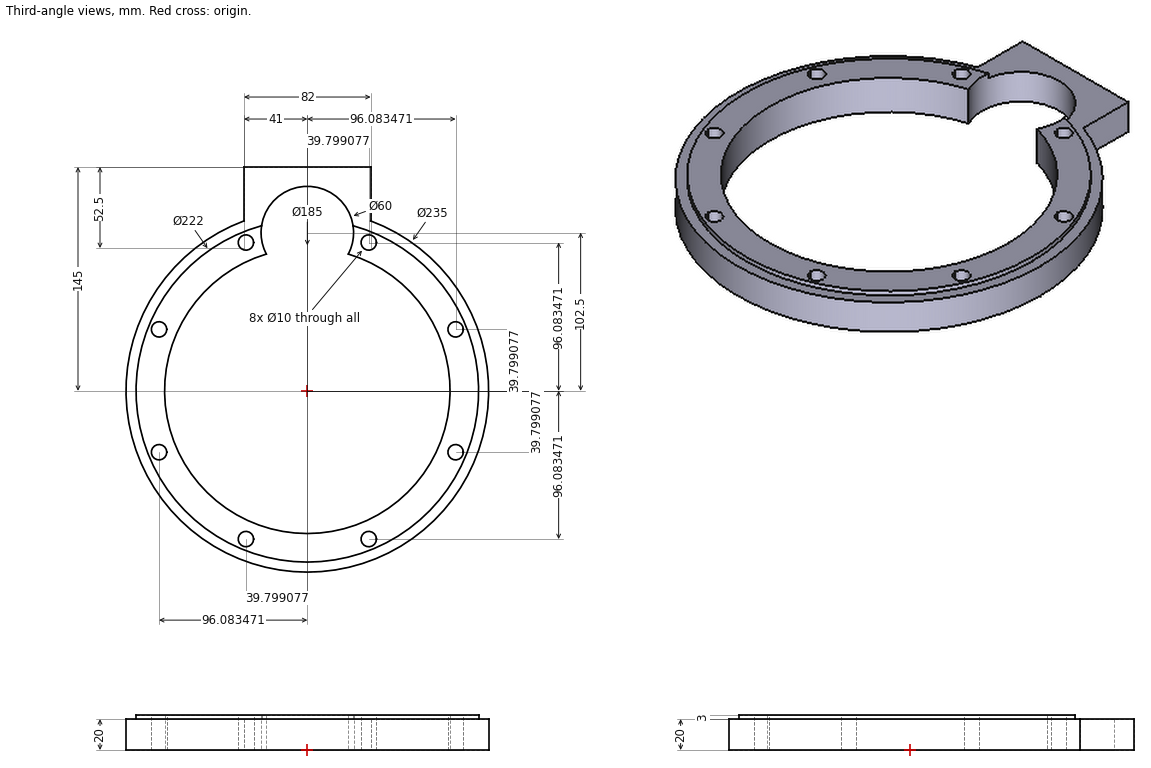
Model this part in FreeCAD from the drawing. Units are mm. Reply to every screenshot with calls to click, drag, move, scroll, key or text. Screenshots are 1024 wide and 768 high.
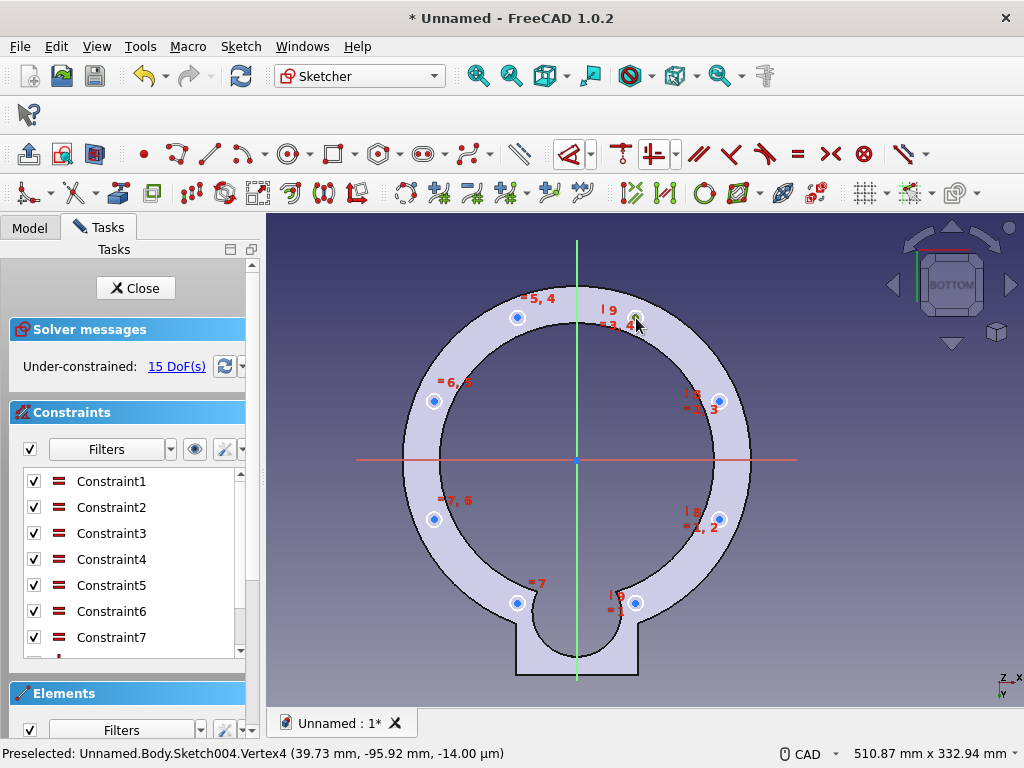
click(518, 318)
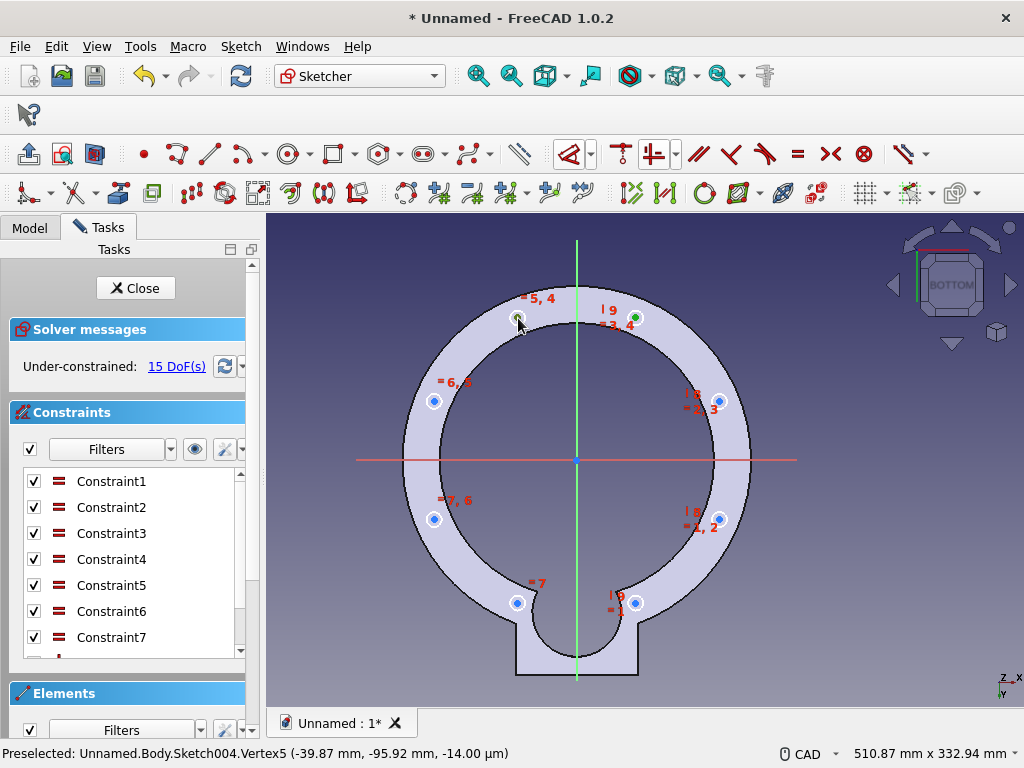
click(676, 154)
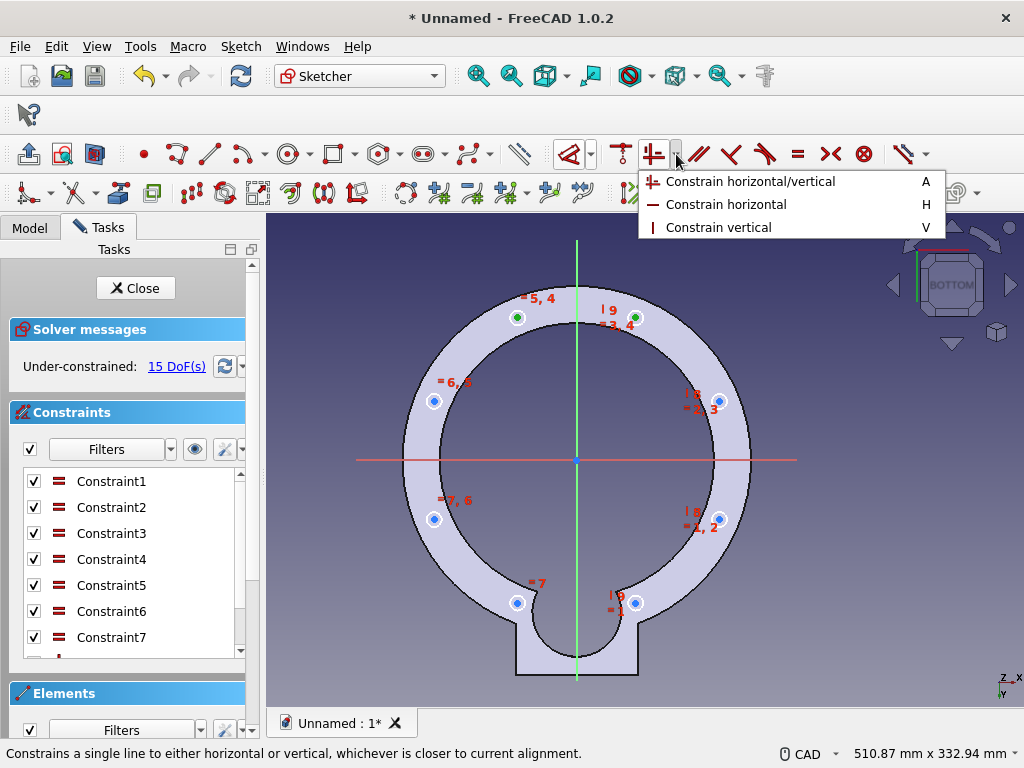
click(792, 204)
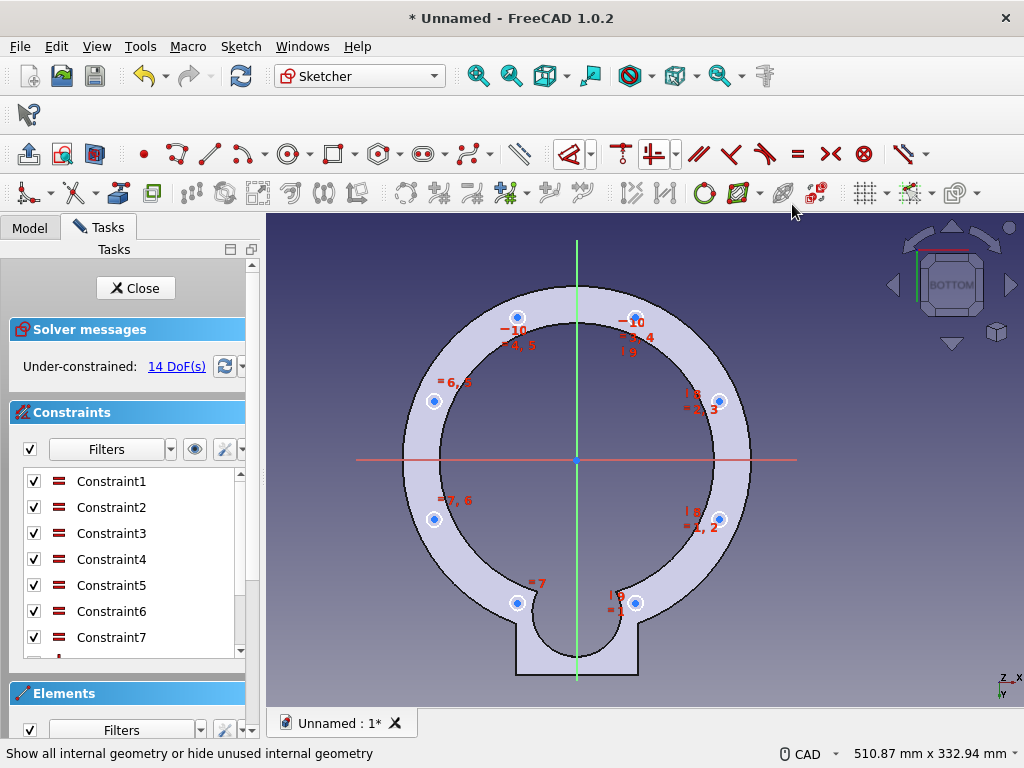
click(719, 401)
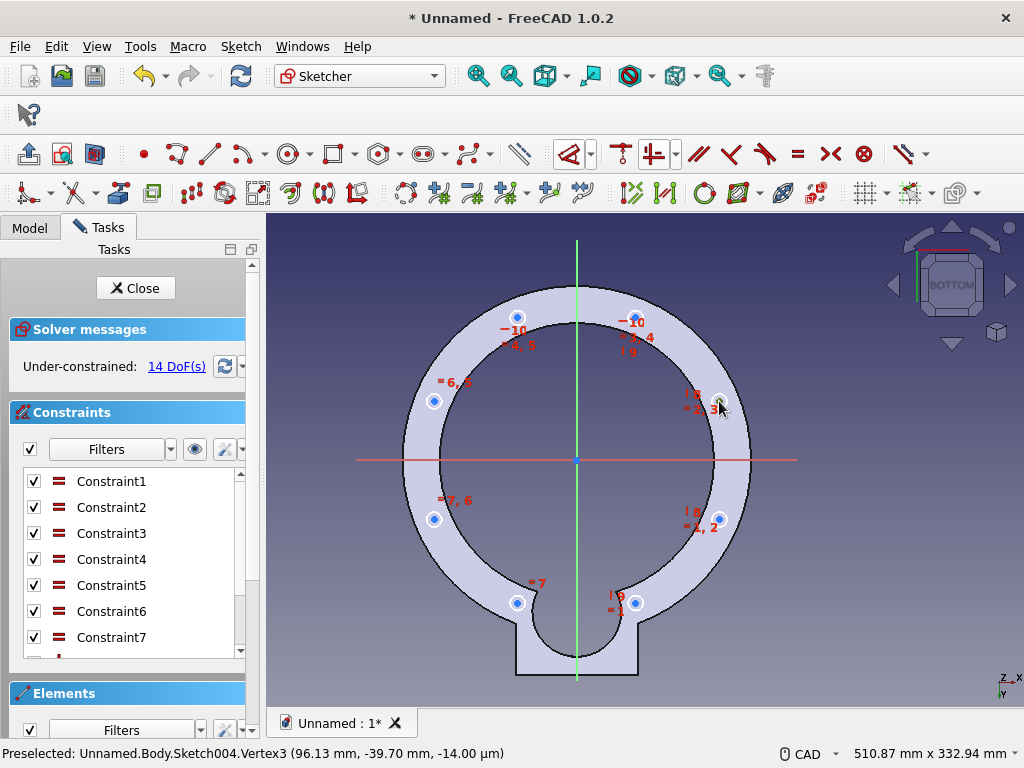
click(434, 401)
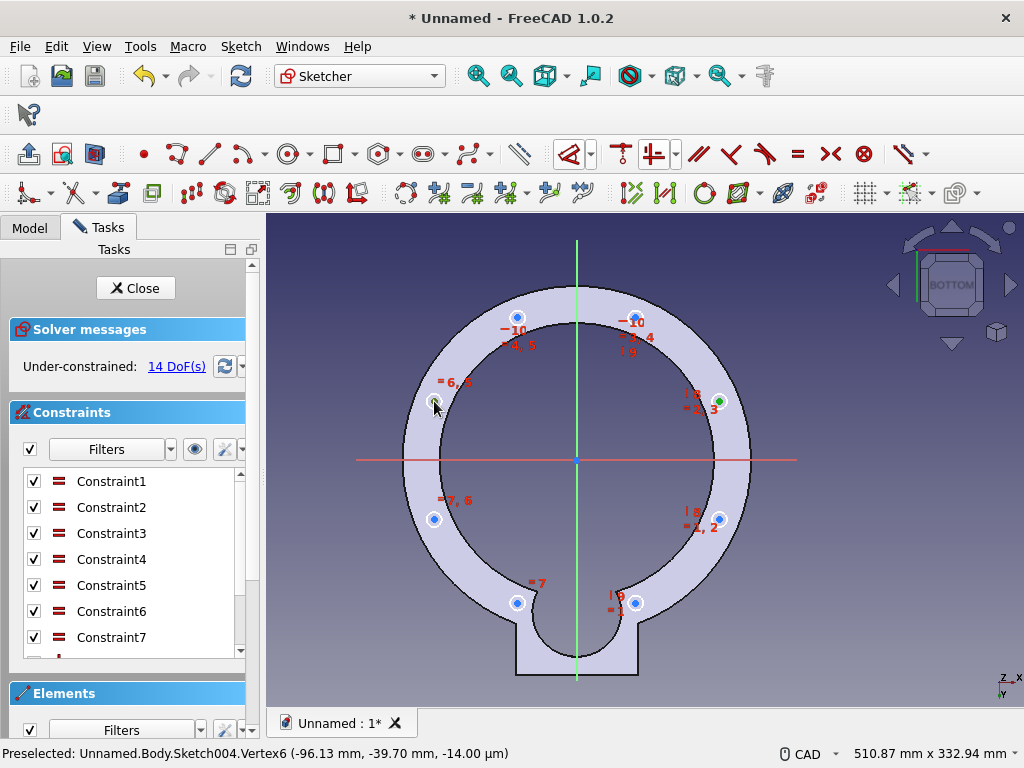
key(h)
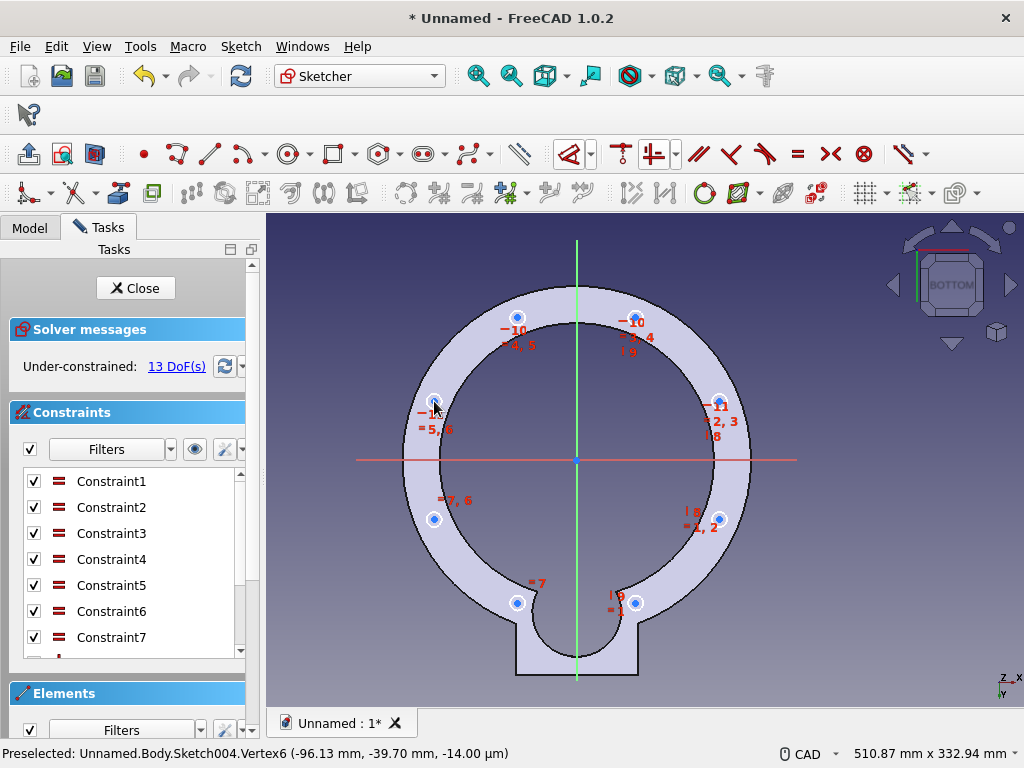
click(434, 401)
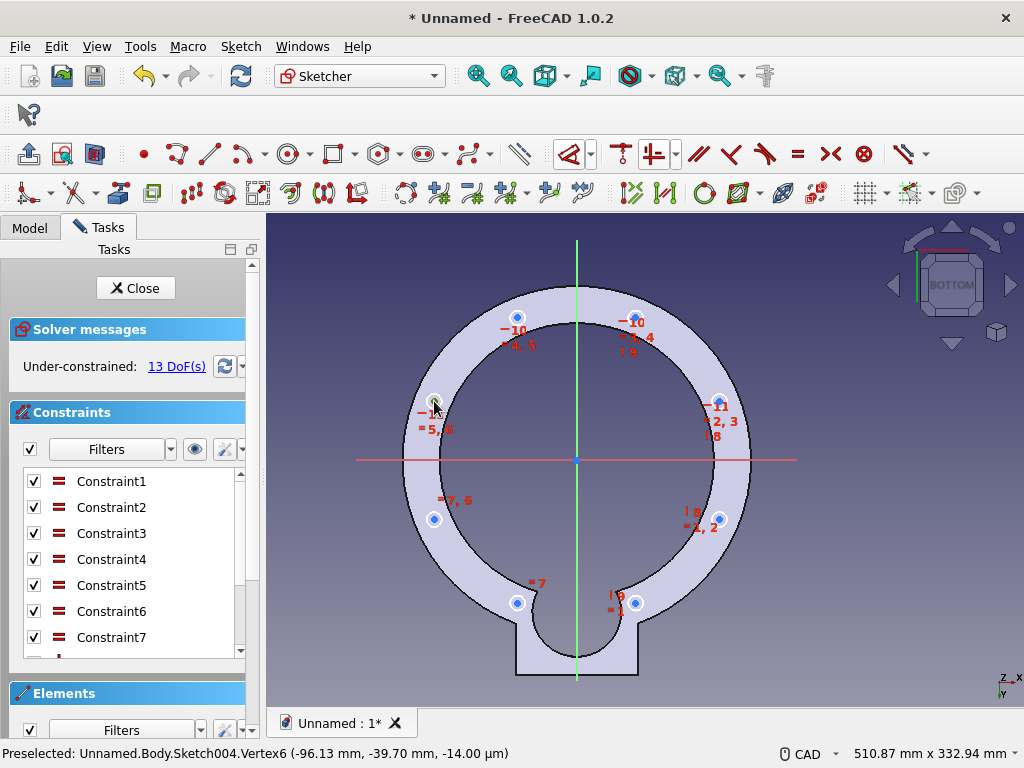
click(434, 520)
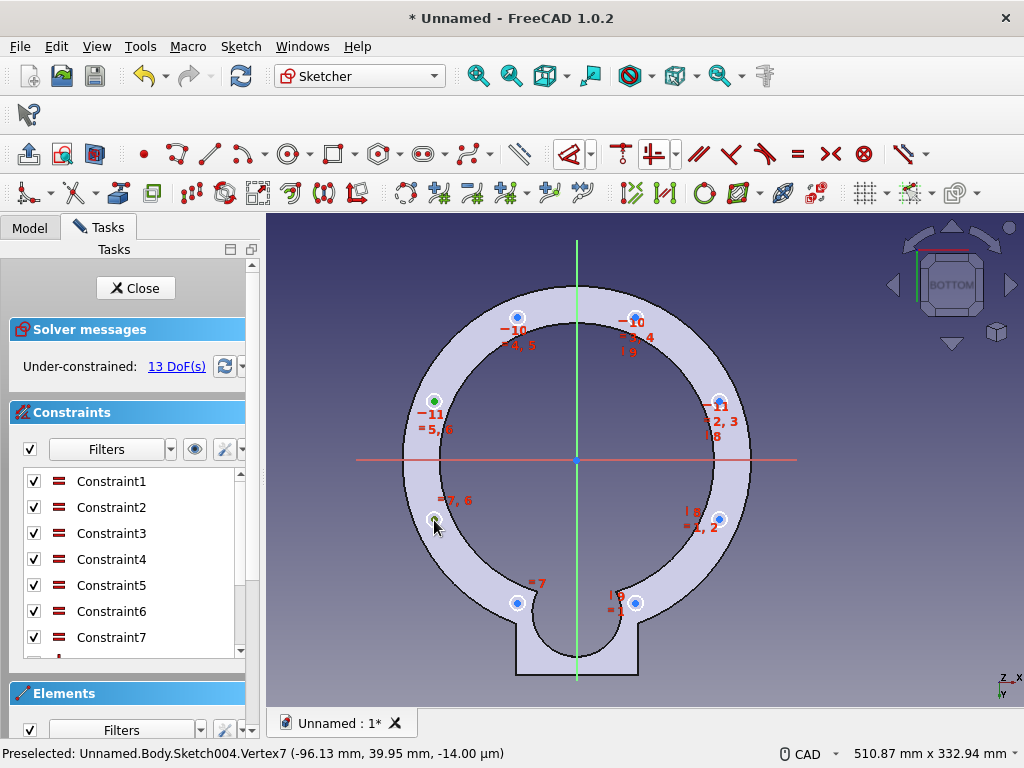
key(v)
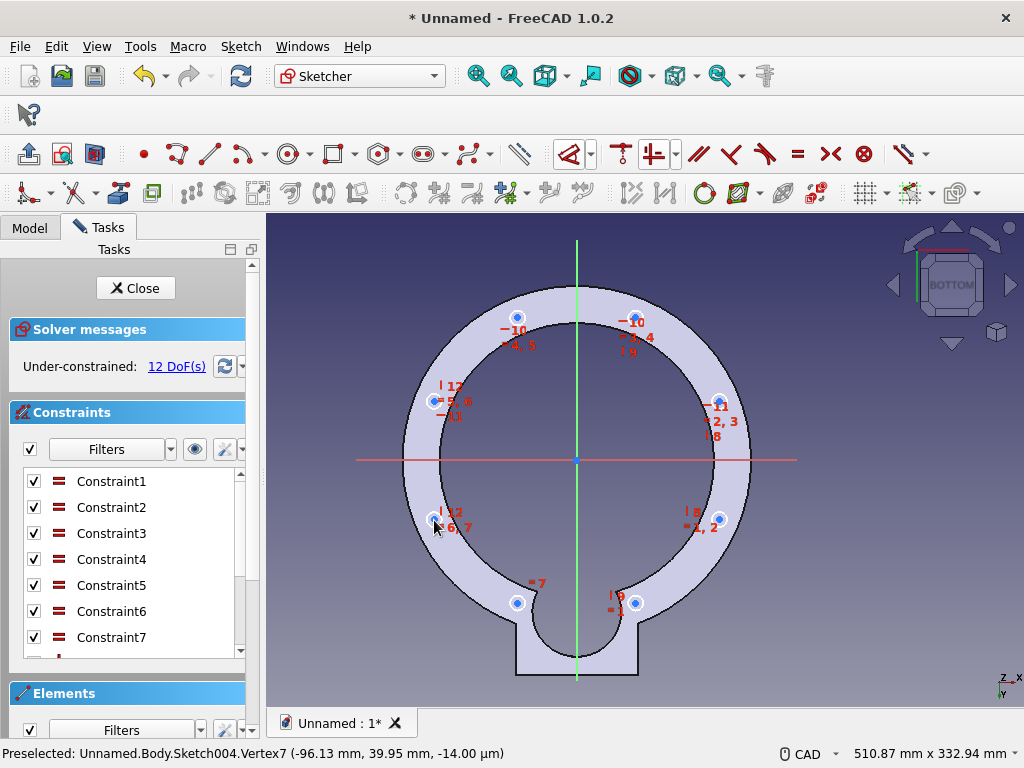
click(719, 520)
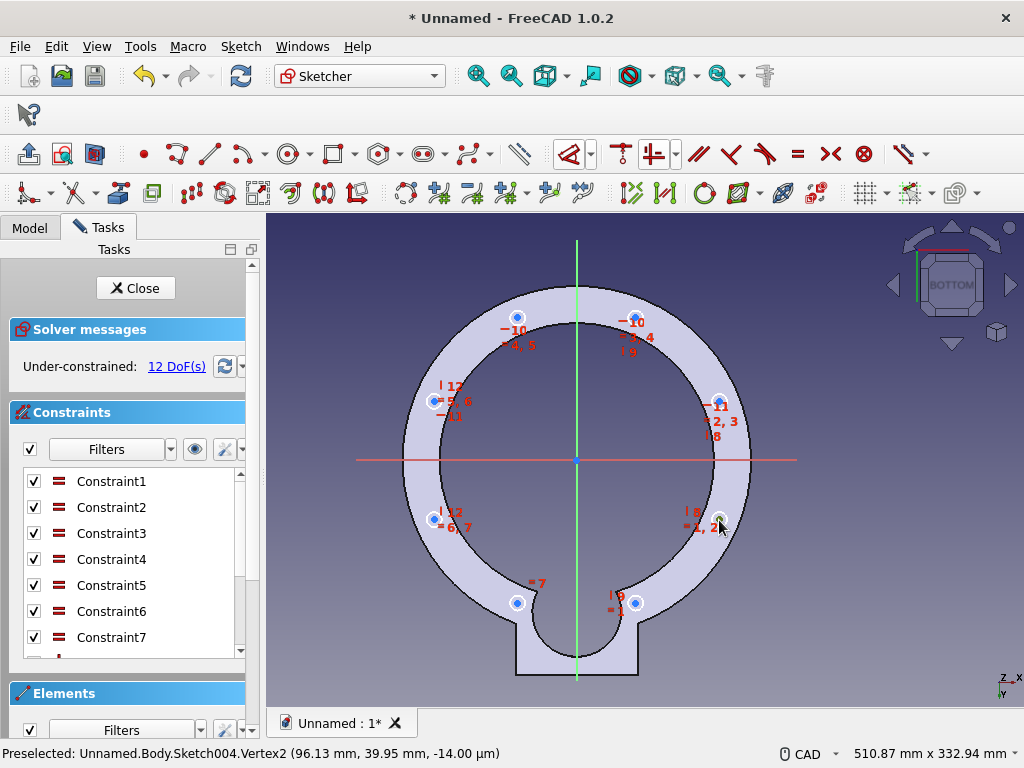
click(434, 520)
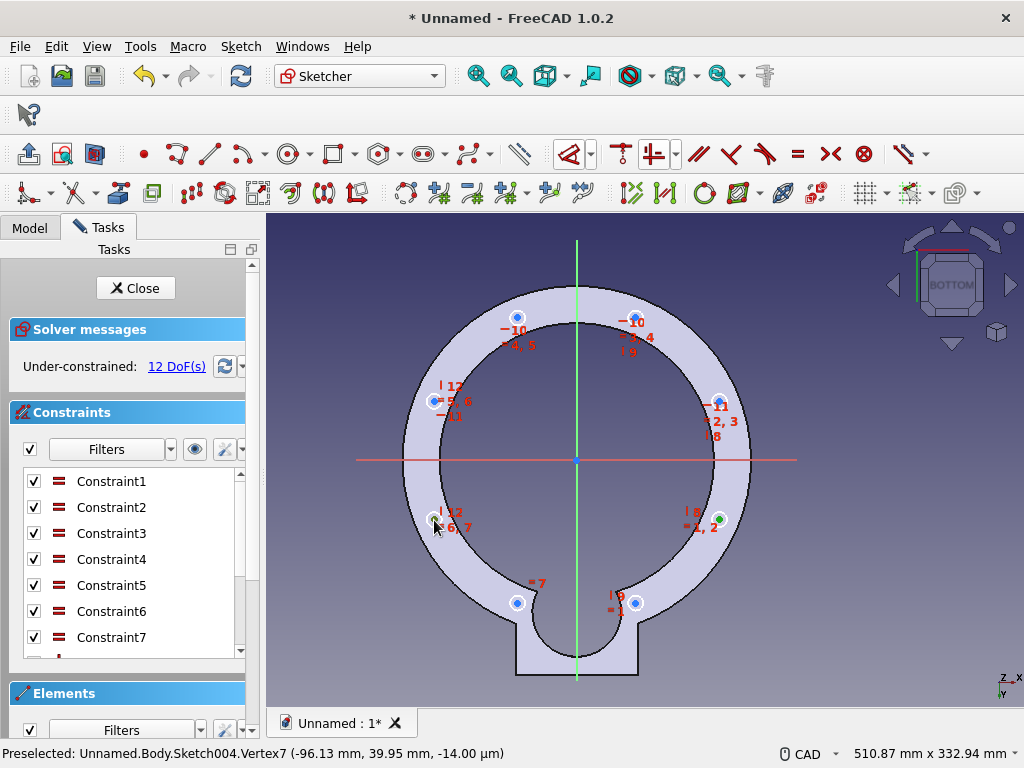
key(h)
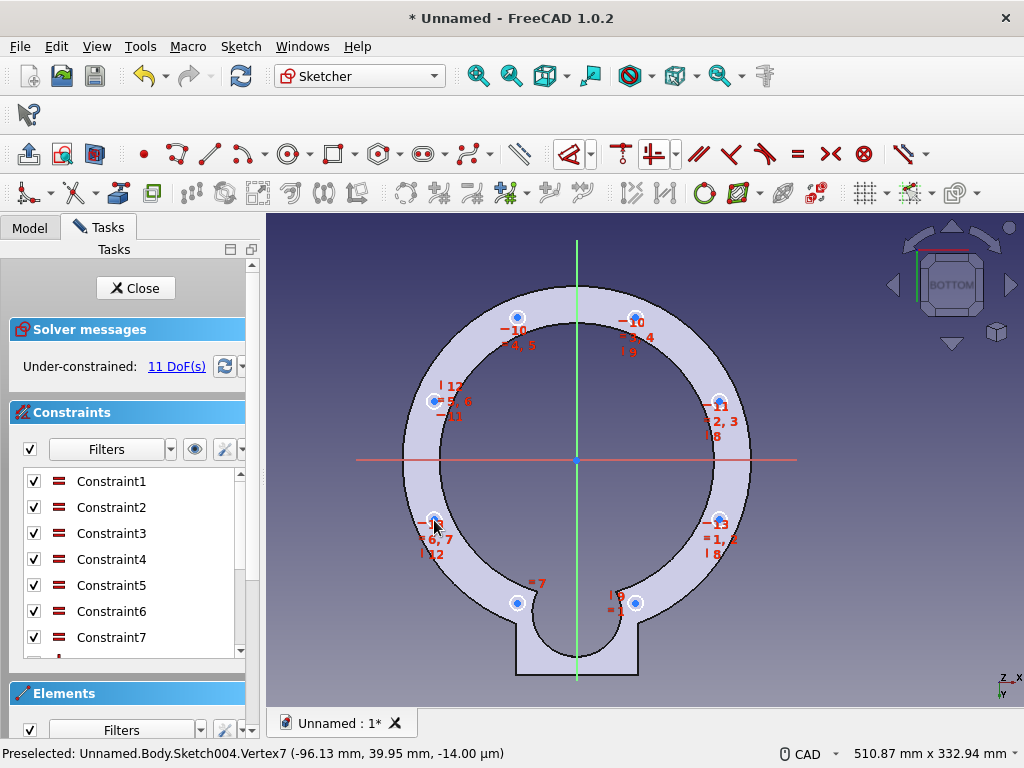
click(518, 318)